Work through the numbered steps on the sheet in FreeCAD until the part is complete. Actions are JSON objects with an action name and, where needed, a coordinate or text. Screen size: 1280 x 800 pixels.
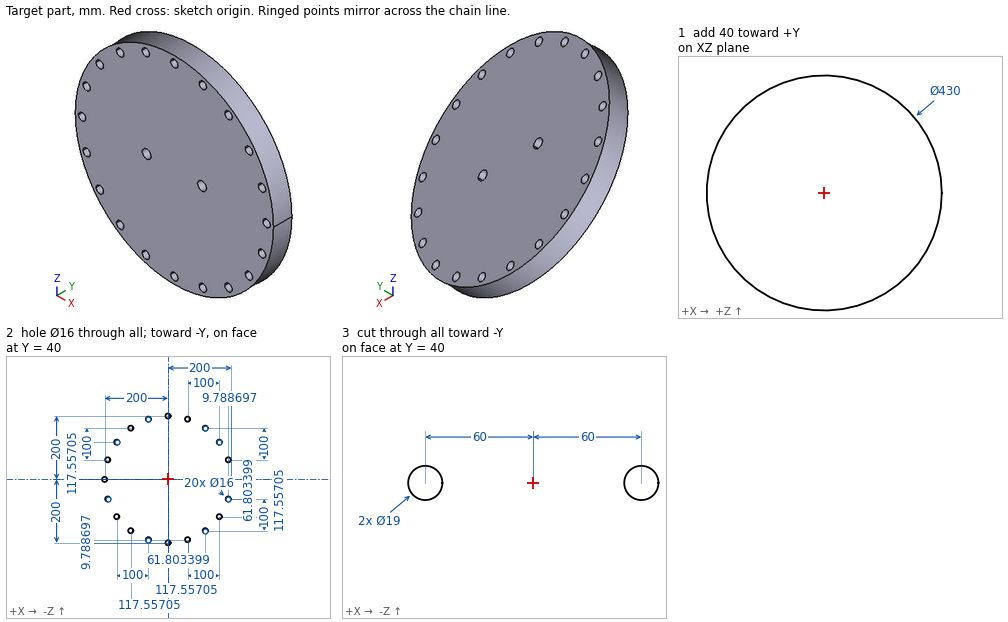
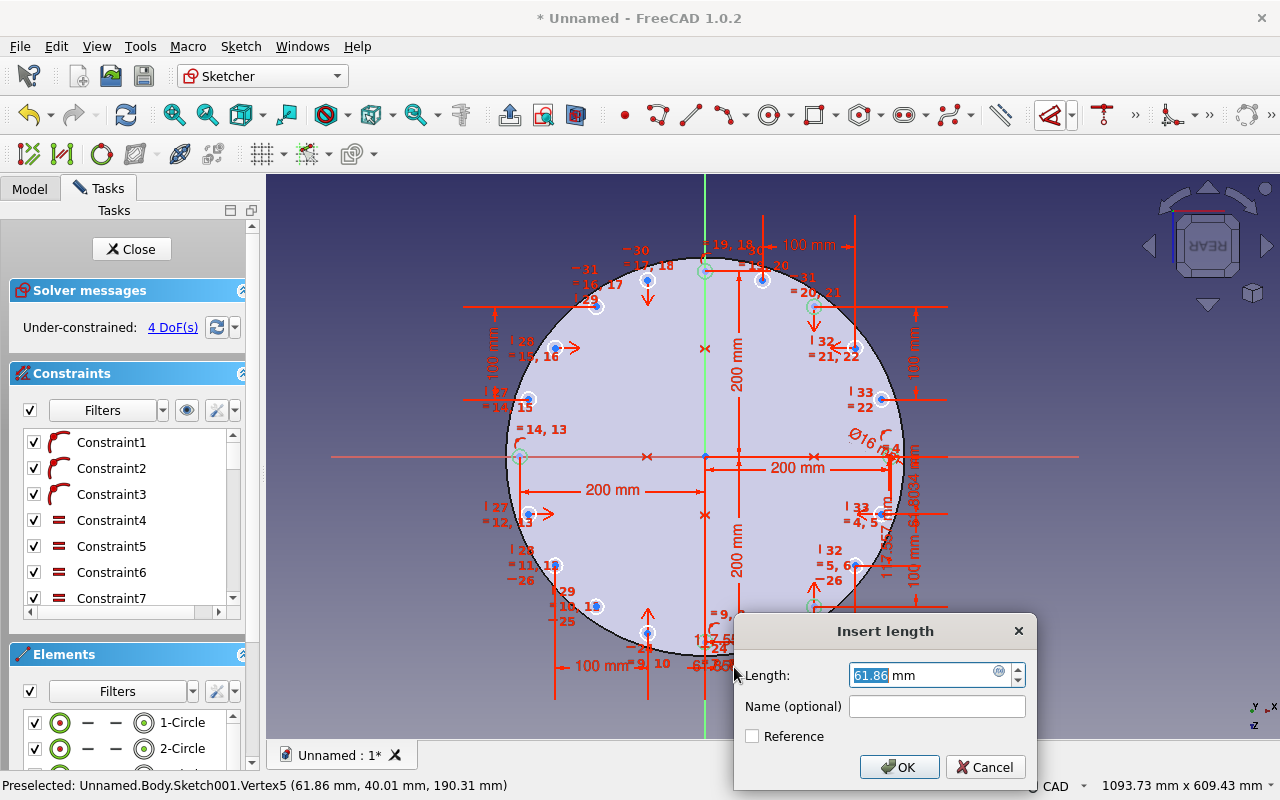
{"action": "type", "text": "61.803399"}
{"action": "key", "text": "Return"}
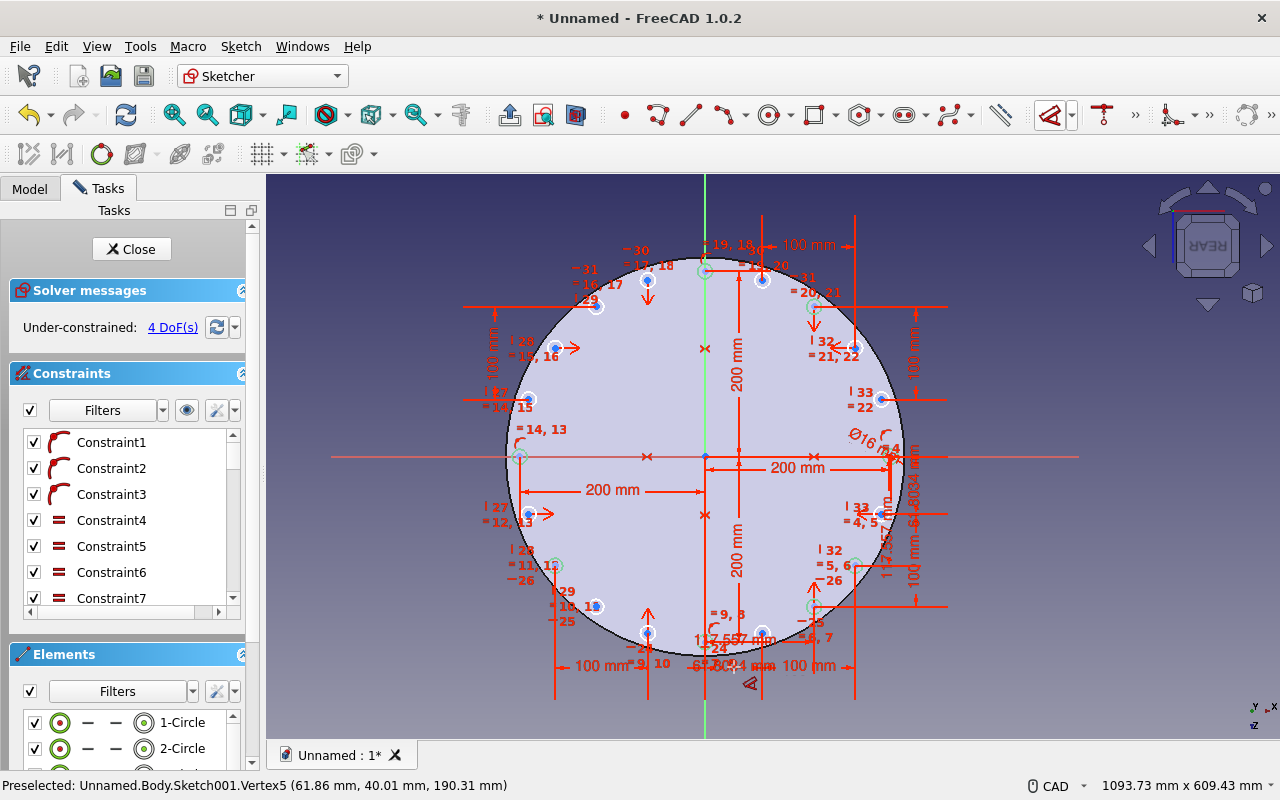
{"action": "left_click", "coordinate": [596, 607]}
{"action": "left_click", "coordinate": [626, 641]}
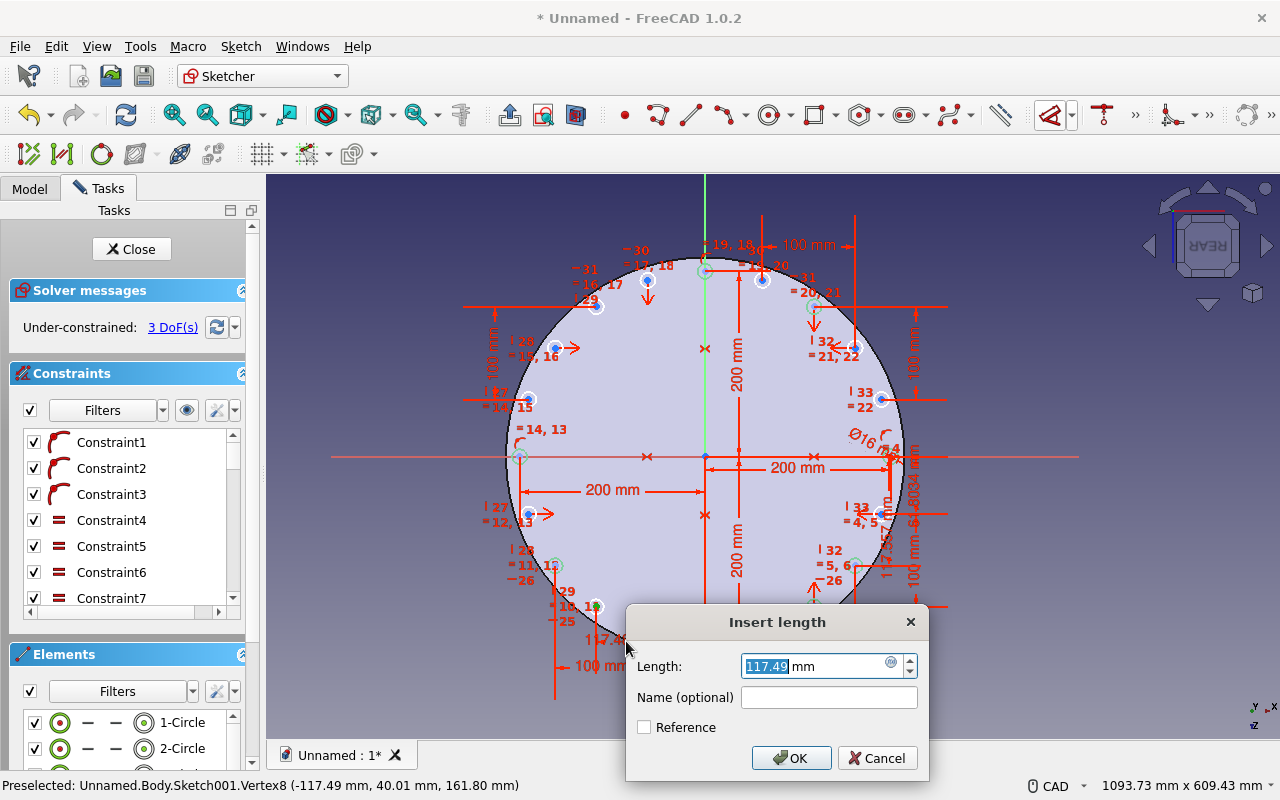
{"action": "type", "text": "117.55705"}
{"action": "key", "text": "Return"}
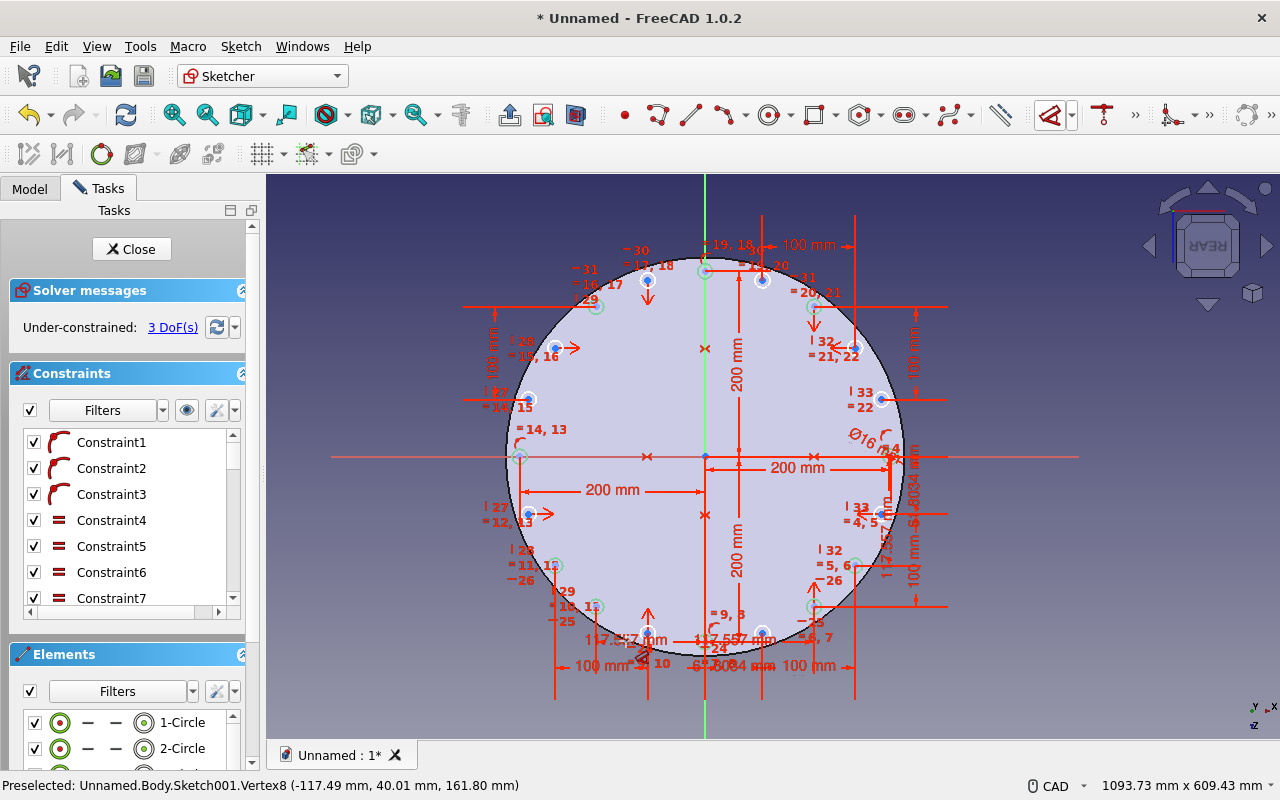
{"action": "left_click", "coordinate": [555, 348]}
{"action": "left_click", "coordinate": [521, 377]}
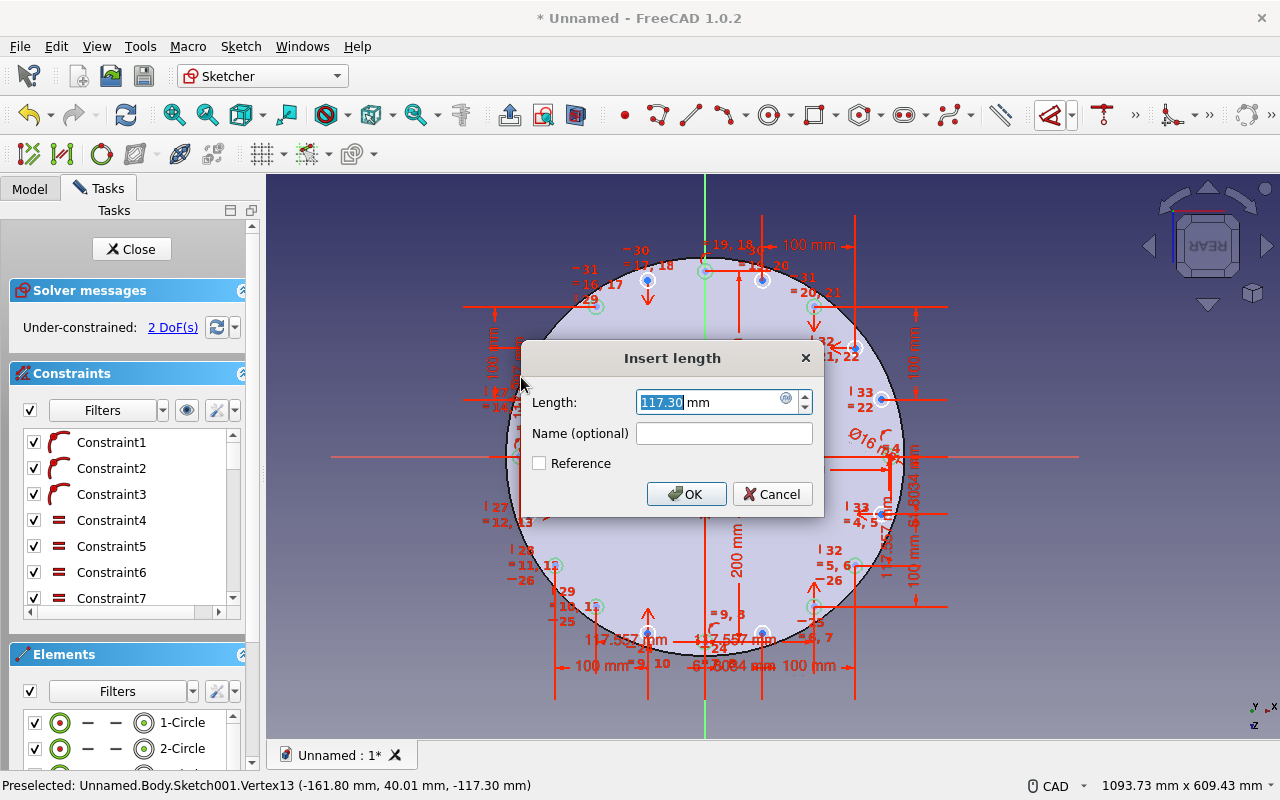
{"action": "type", "text": "117.55705"}
{"action": "key", "text": "Return"}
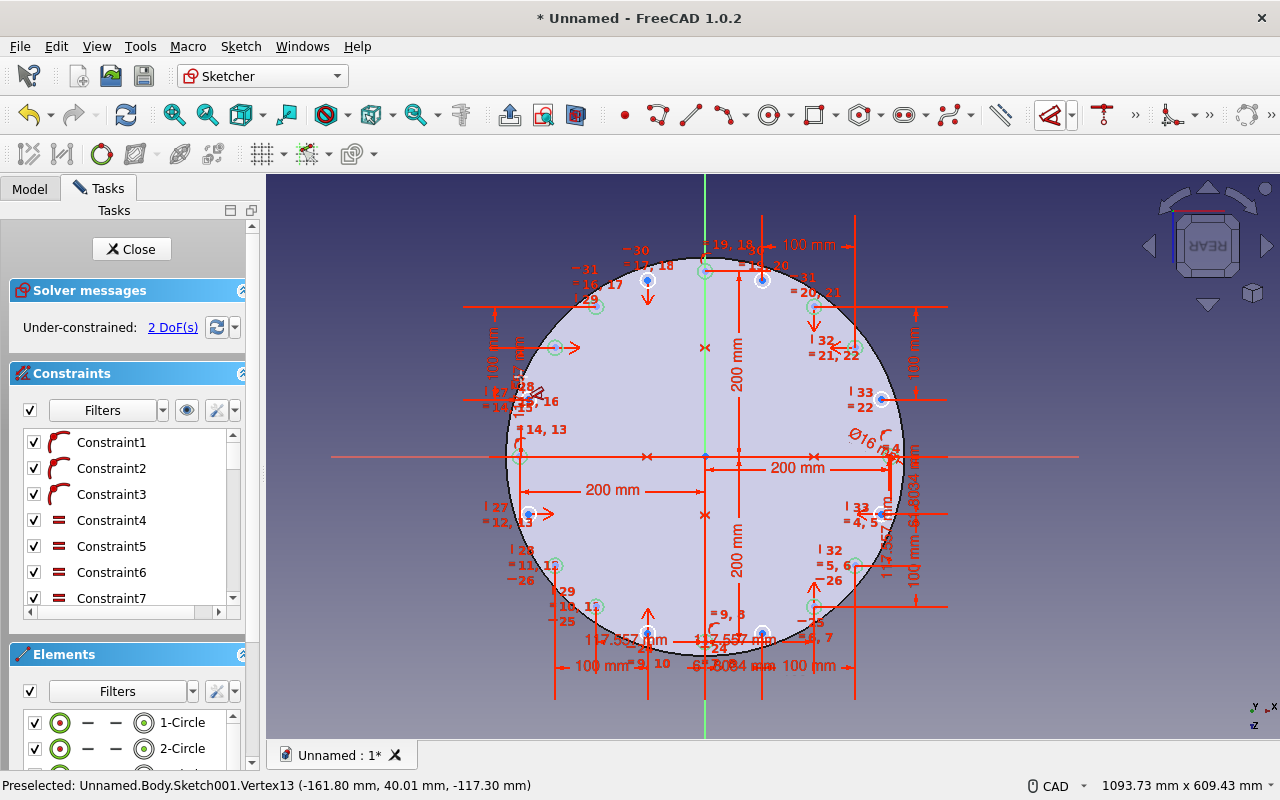
{"action": "scroll", "coordinate": [891, 457], "scroll_direction": "up", "scroll_amount": 8}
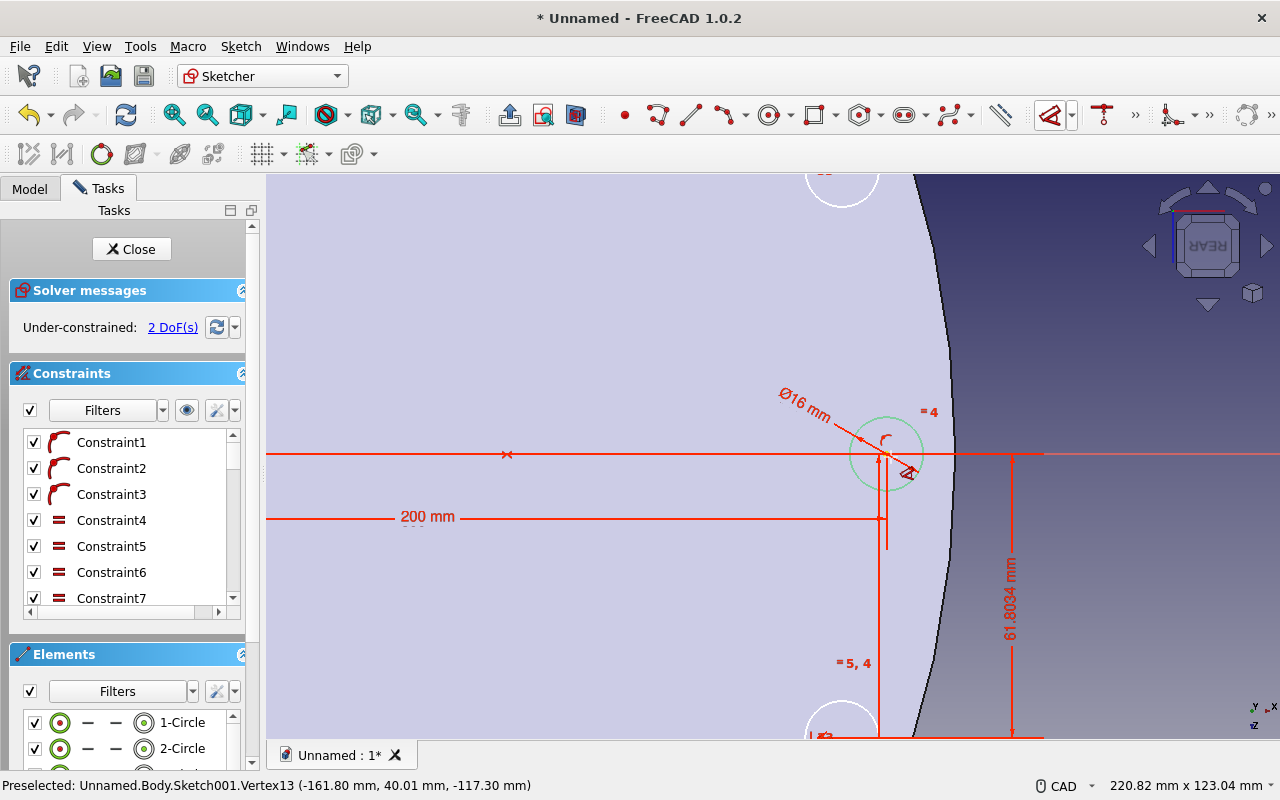
{"action": "left_click", "coordinate": [887, 454]}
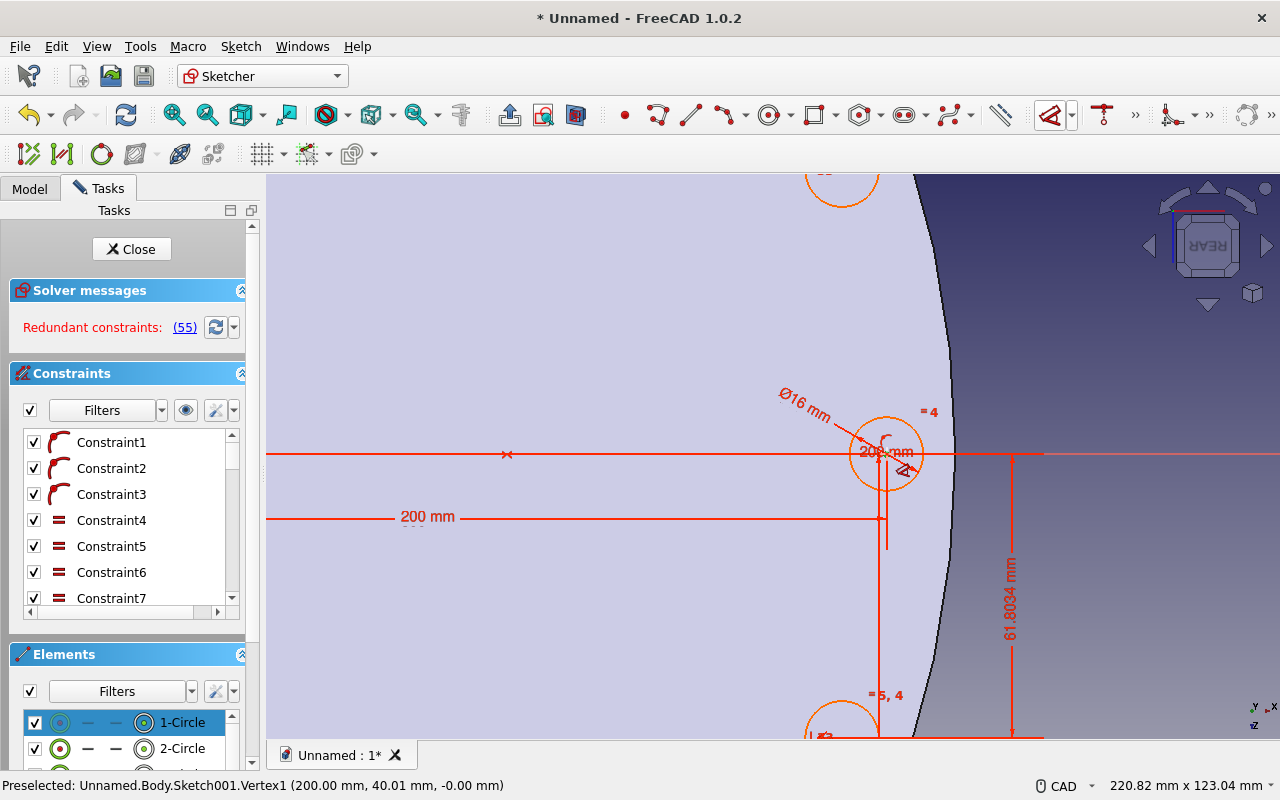
{"action": "scroll", "coordinate": [891, 457], "scroll_direction": "down", "scroll_amount": 8}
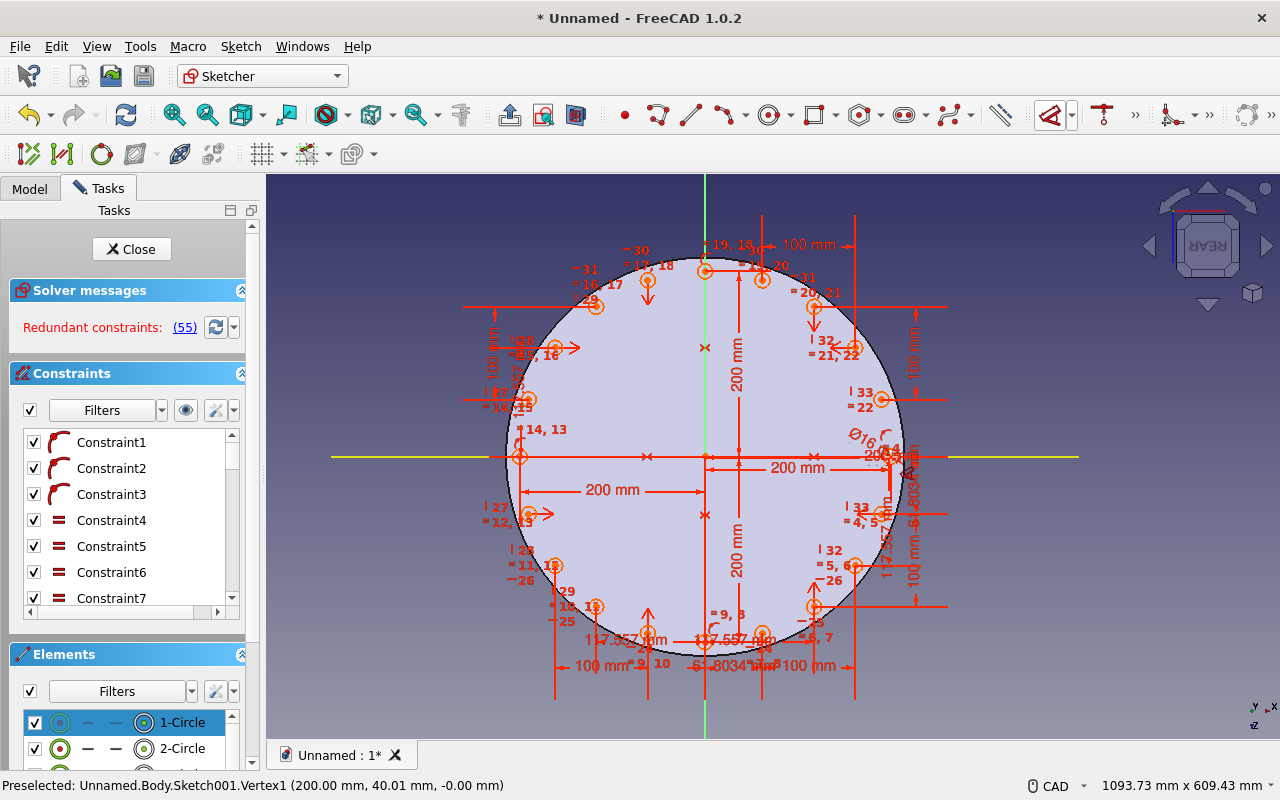
{"action": "scroll", "coordinate": [882, 514], "scroll_direction": "up", "scroll_amount": 8}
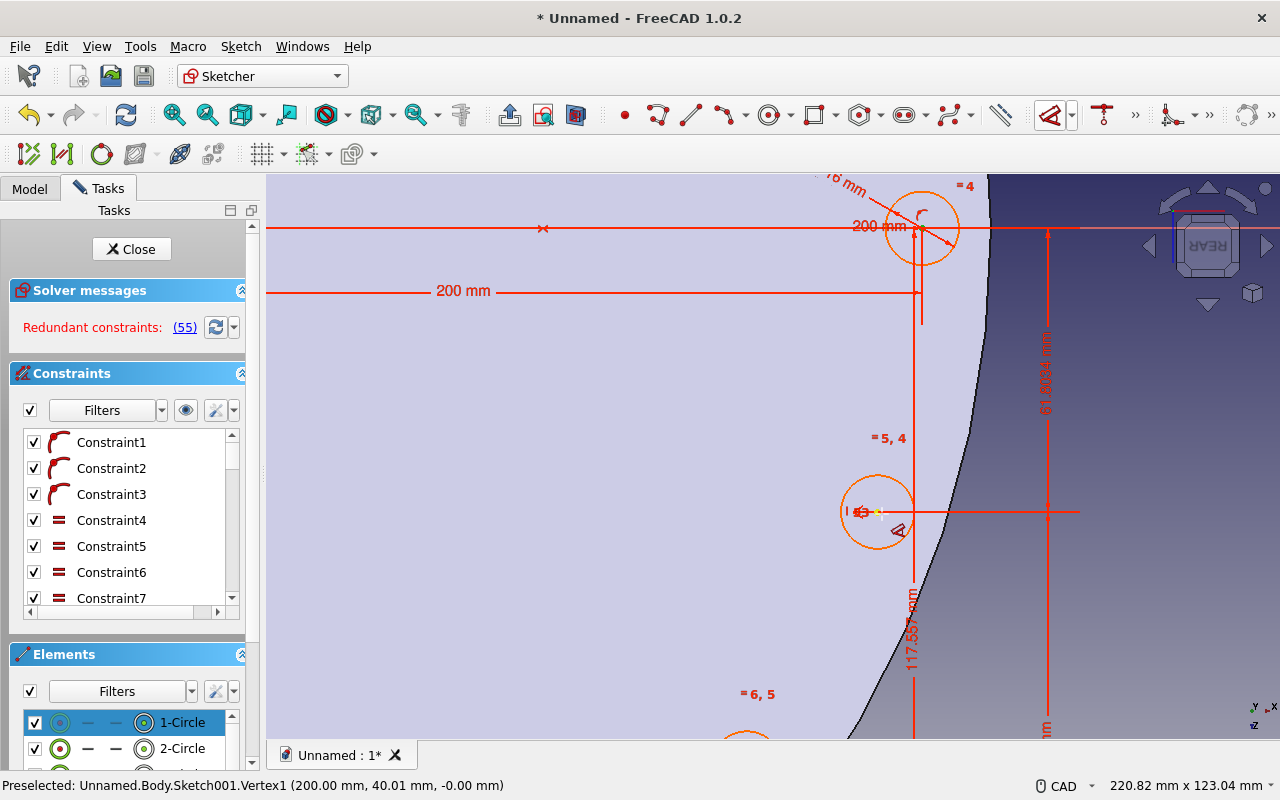
{"action": "left_click", "coordinate": [878, 512]}
{"action": "left_click", "coordinate": [916, 546]}